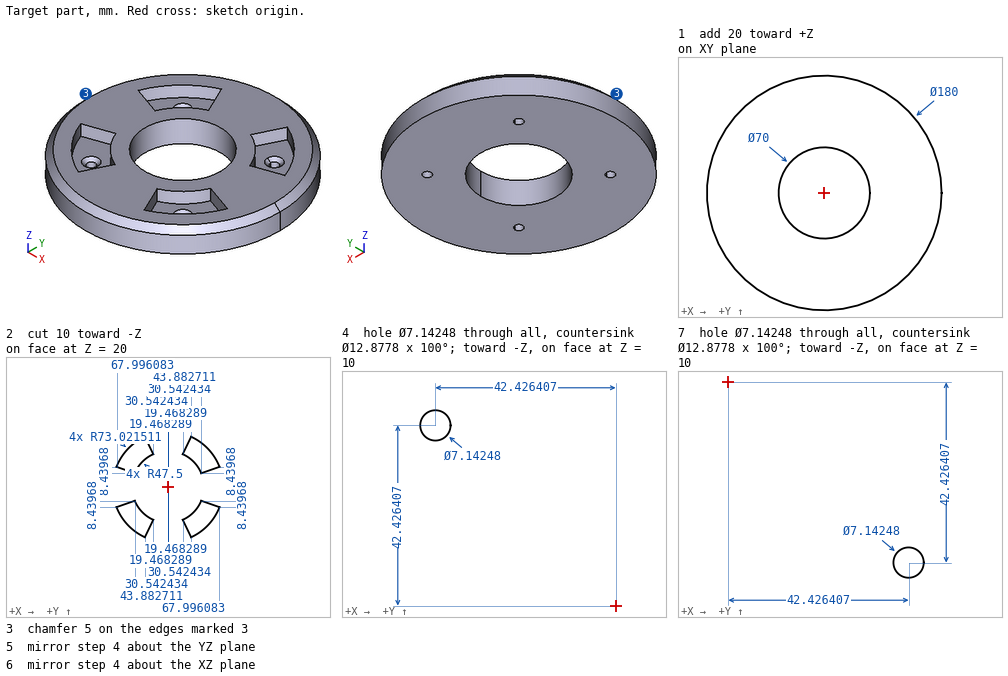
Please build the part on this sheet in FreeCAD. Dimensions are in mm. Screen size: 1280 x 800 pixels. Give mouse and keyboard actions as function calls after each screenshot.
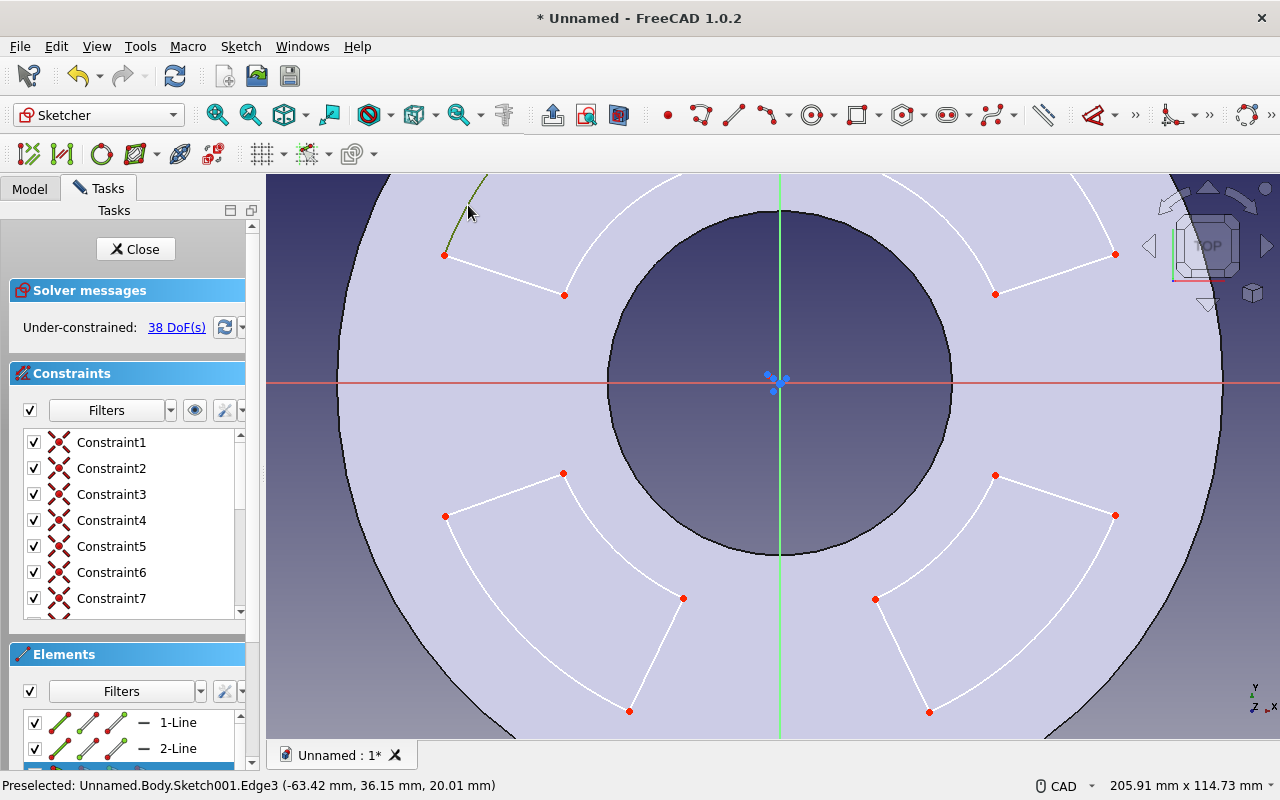
click(1091, 205)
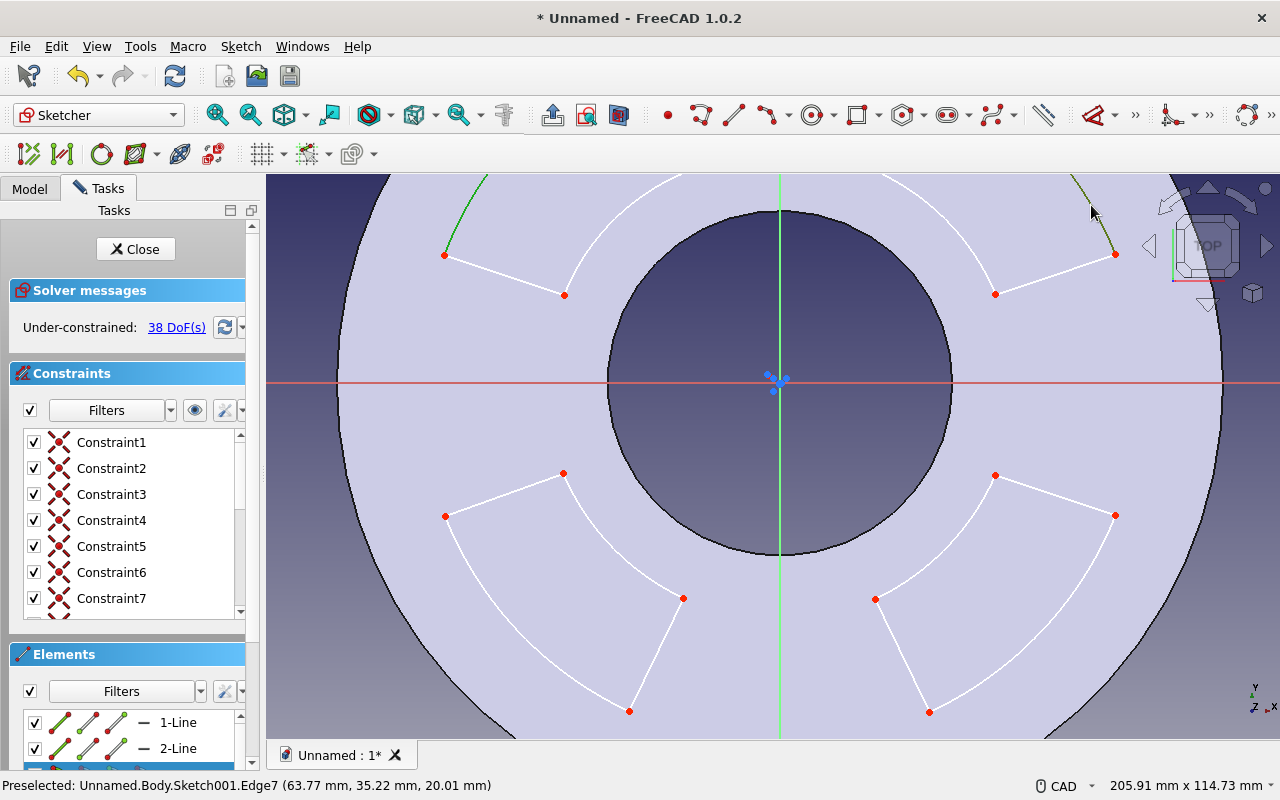
key(c)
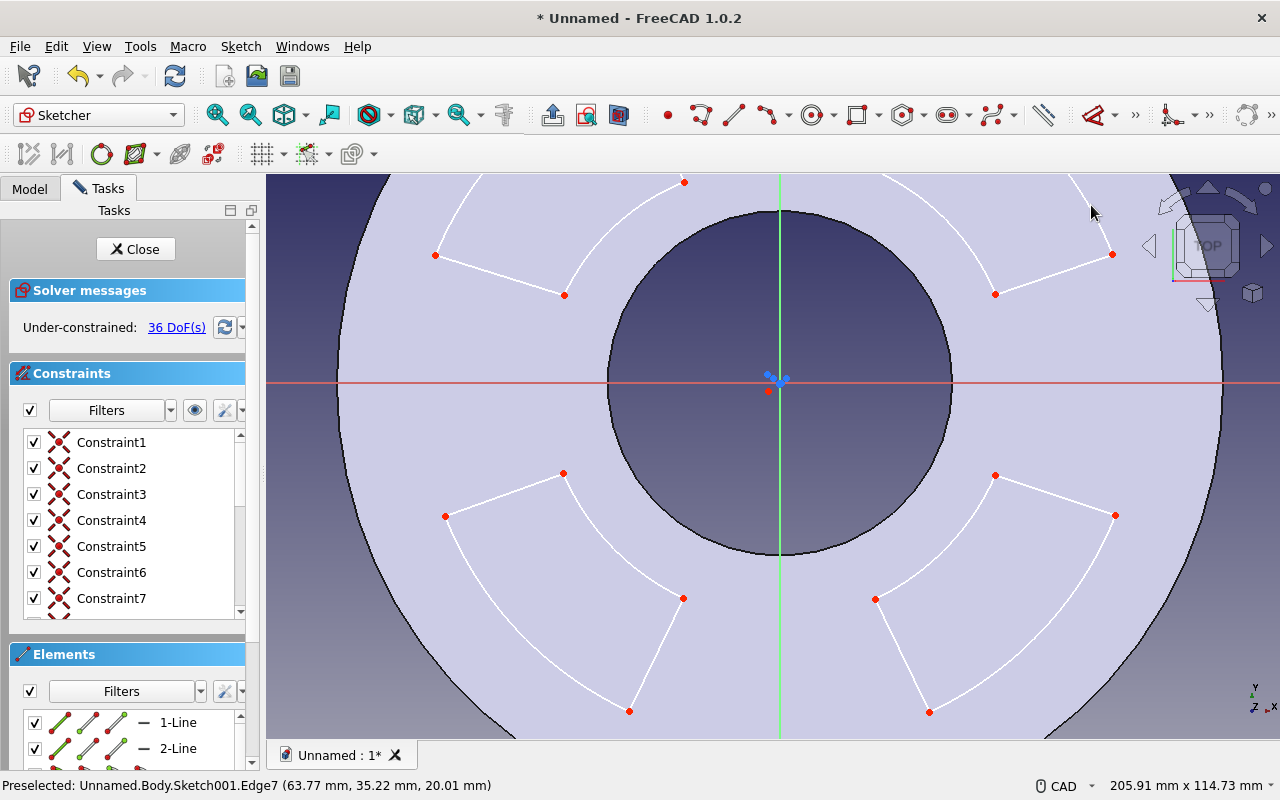
click(461, 205)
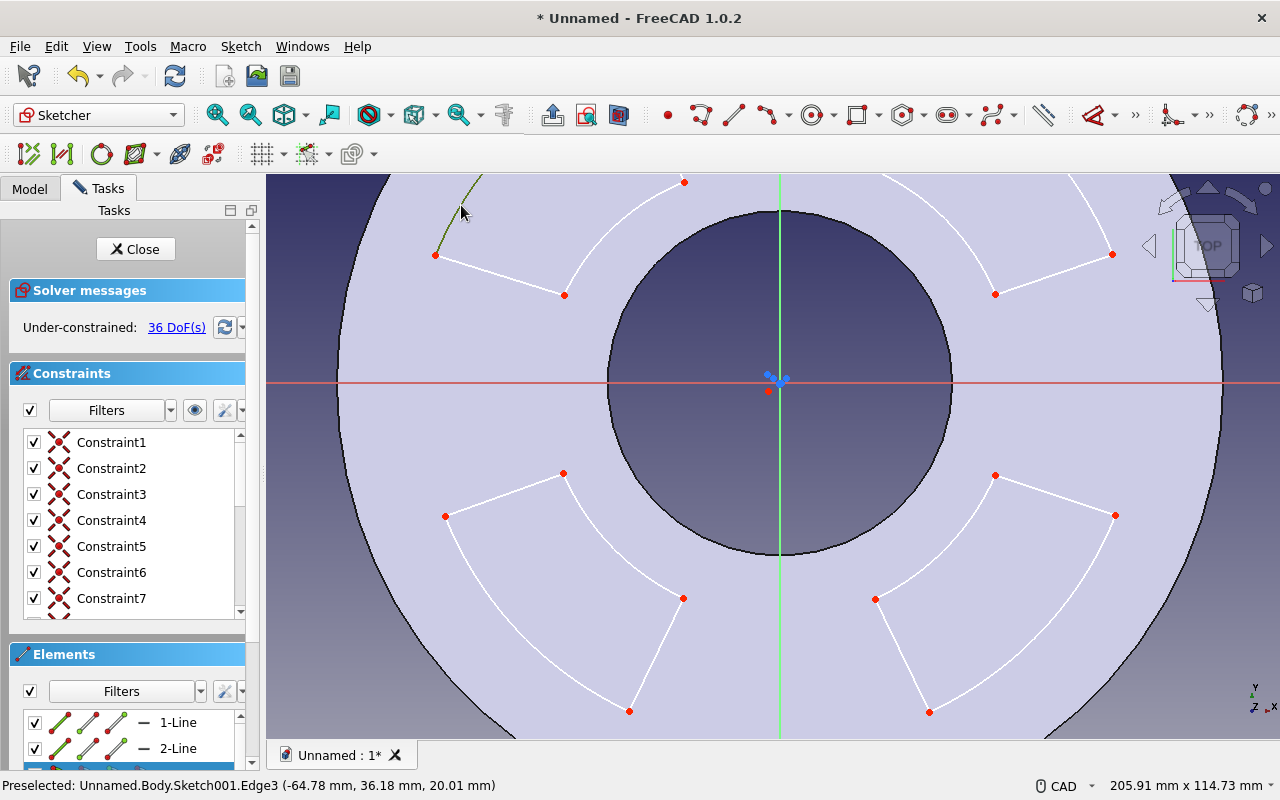
click(970, 248)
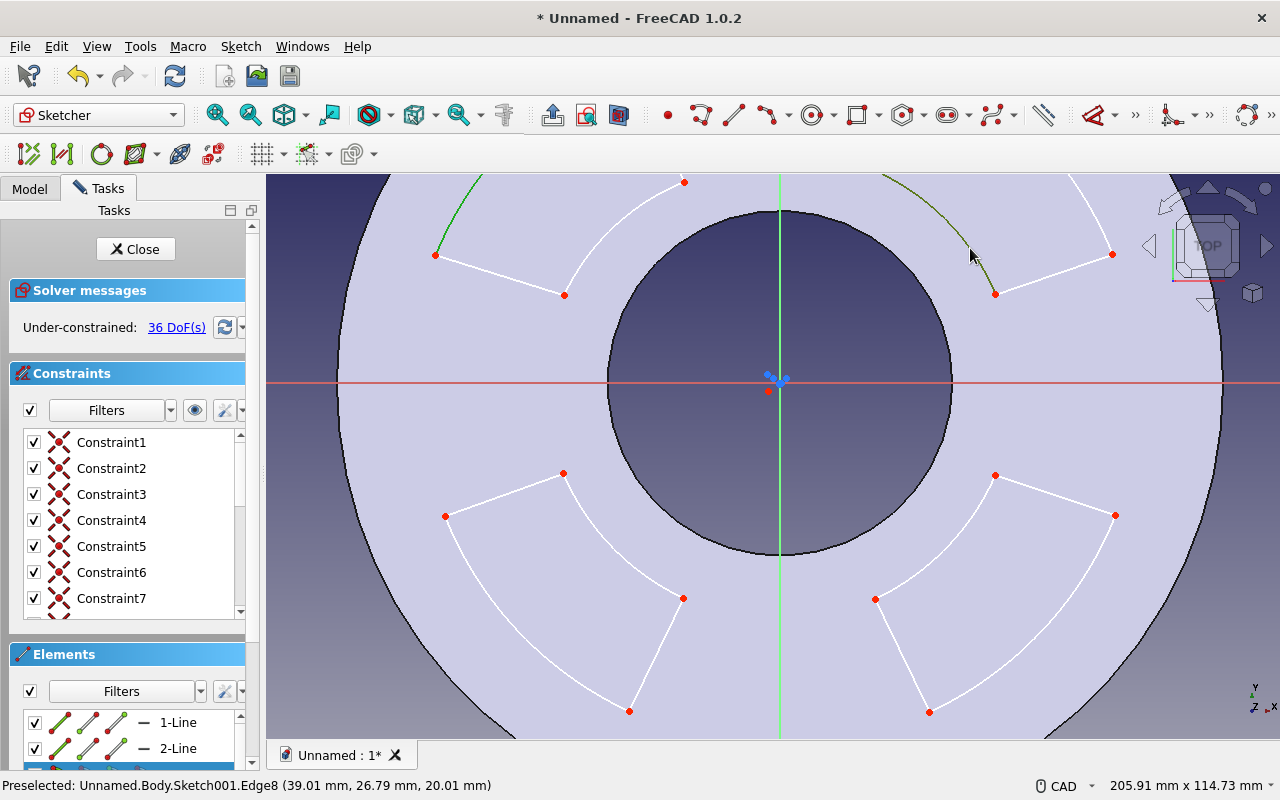
key(c)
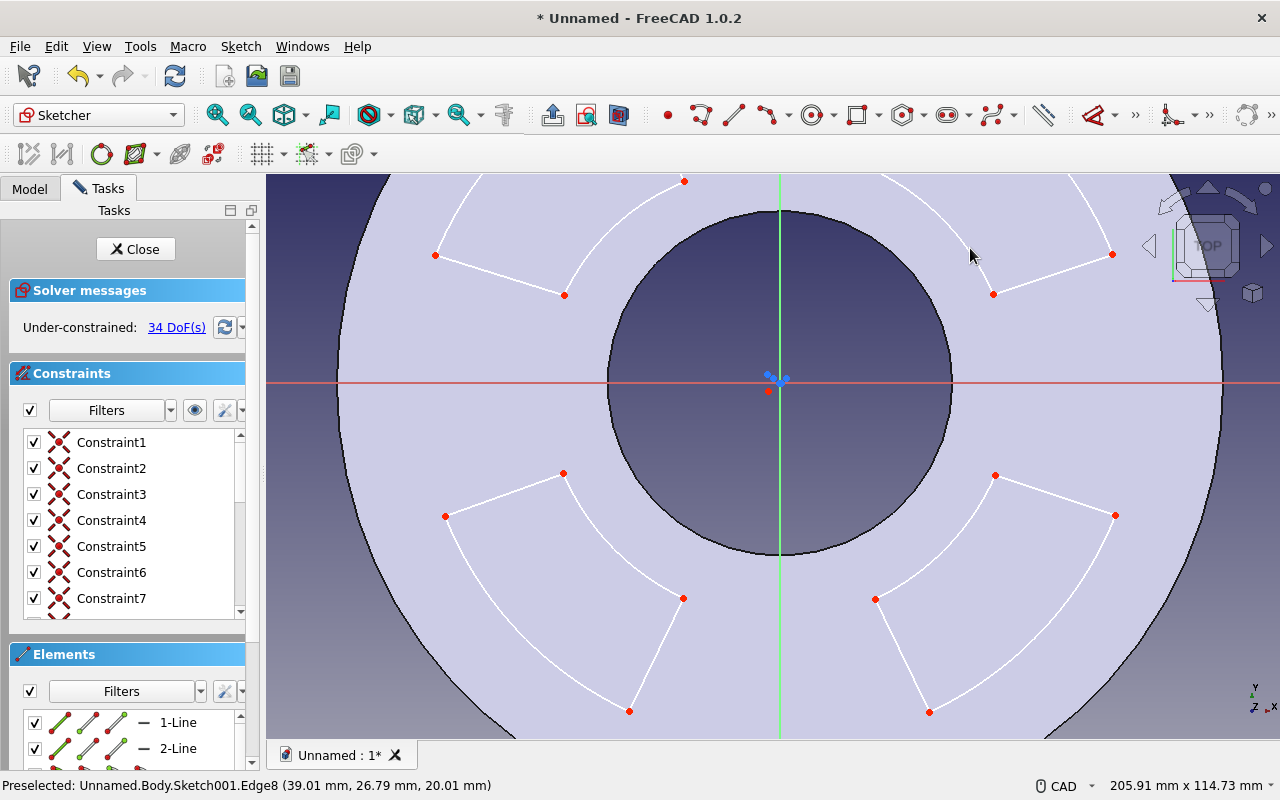
click(461, 205)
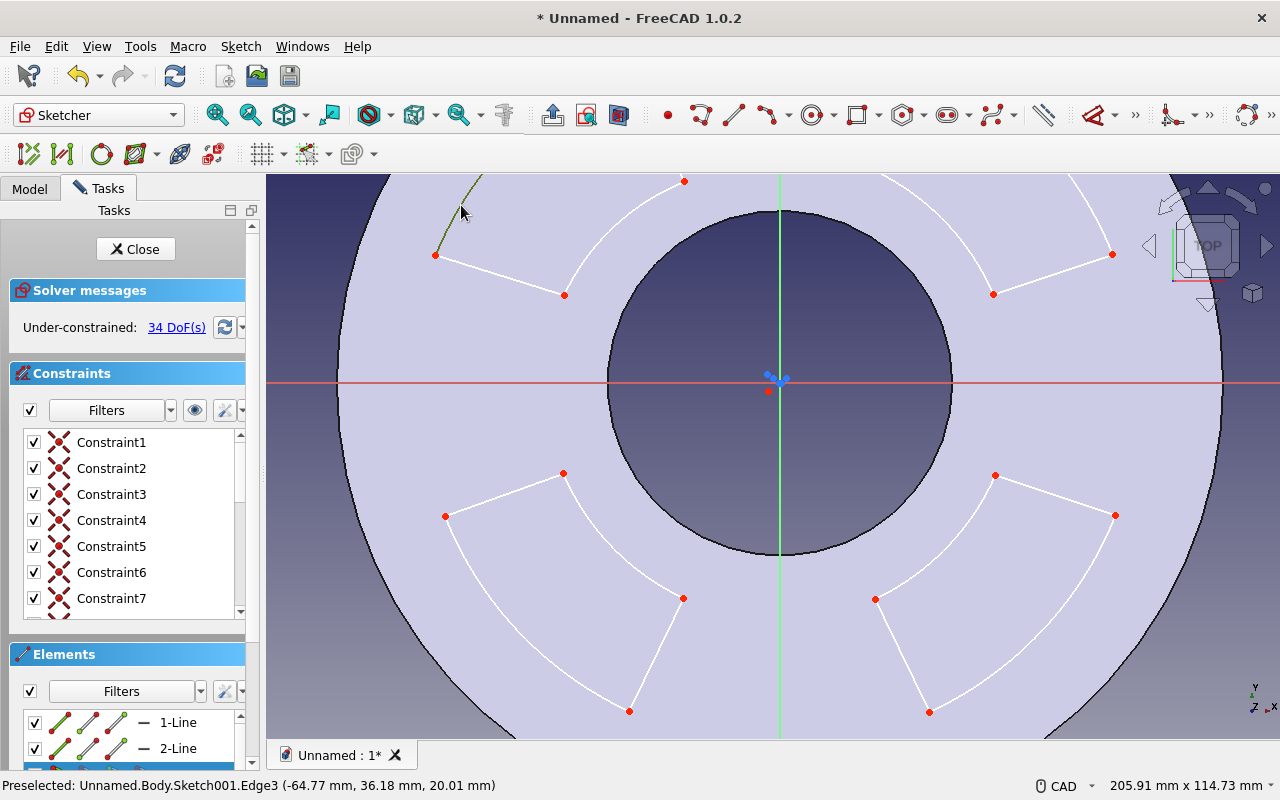
click(1000, 669)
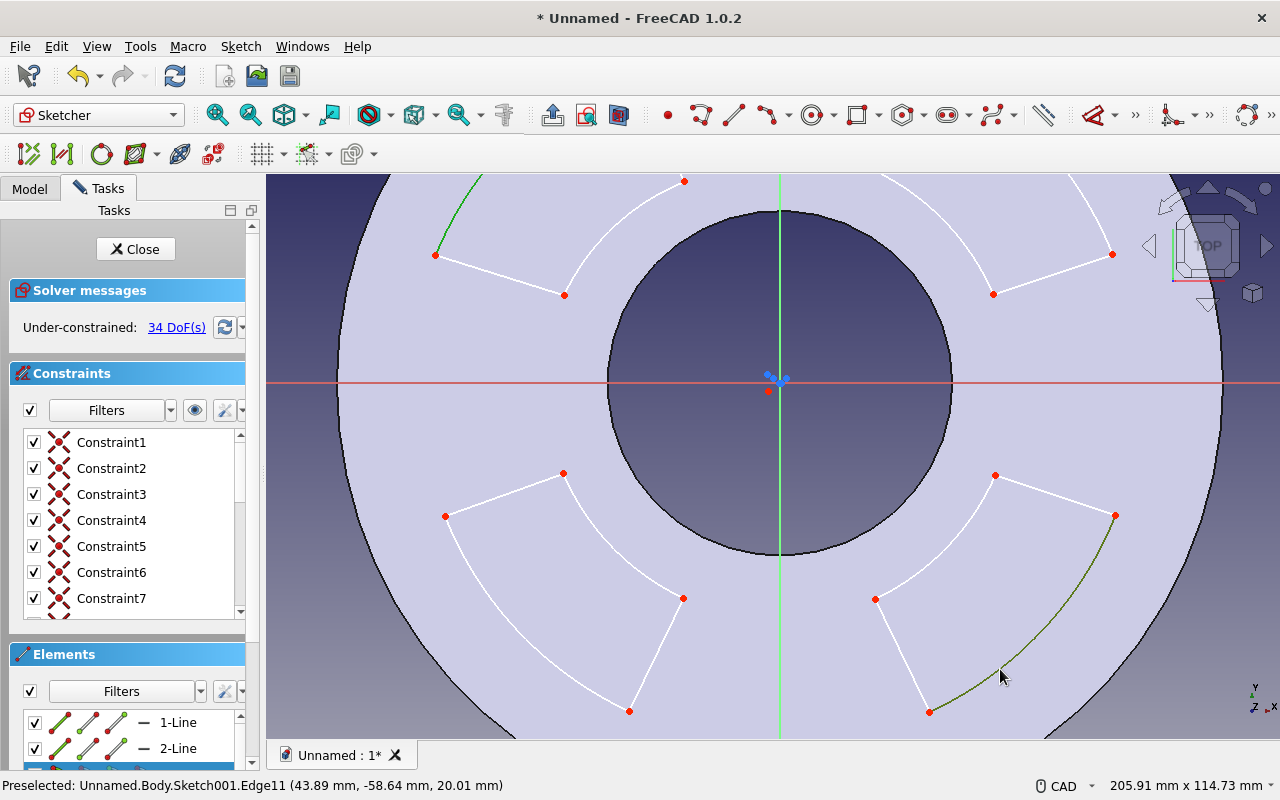
key(c)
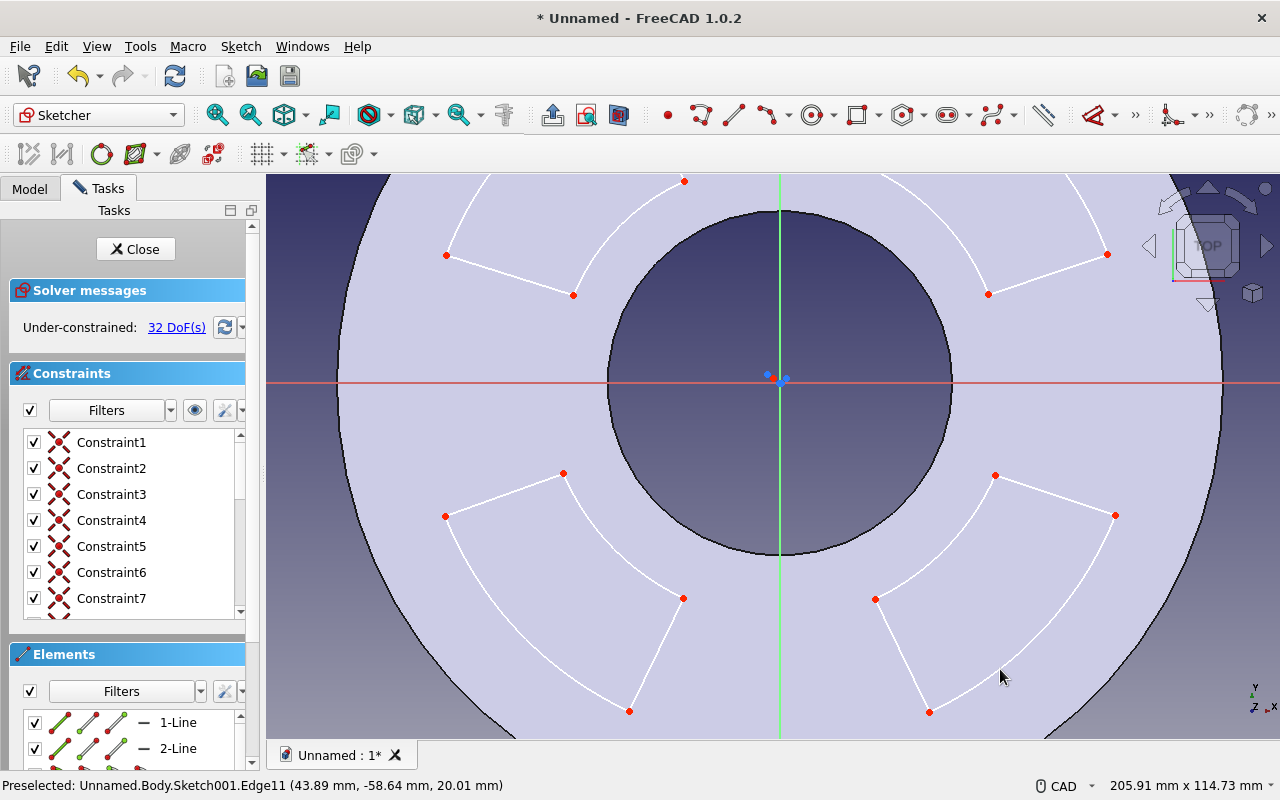
click(470, 206)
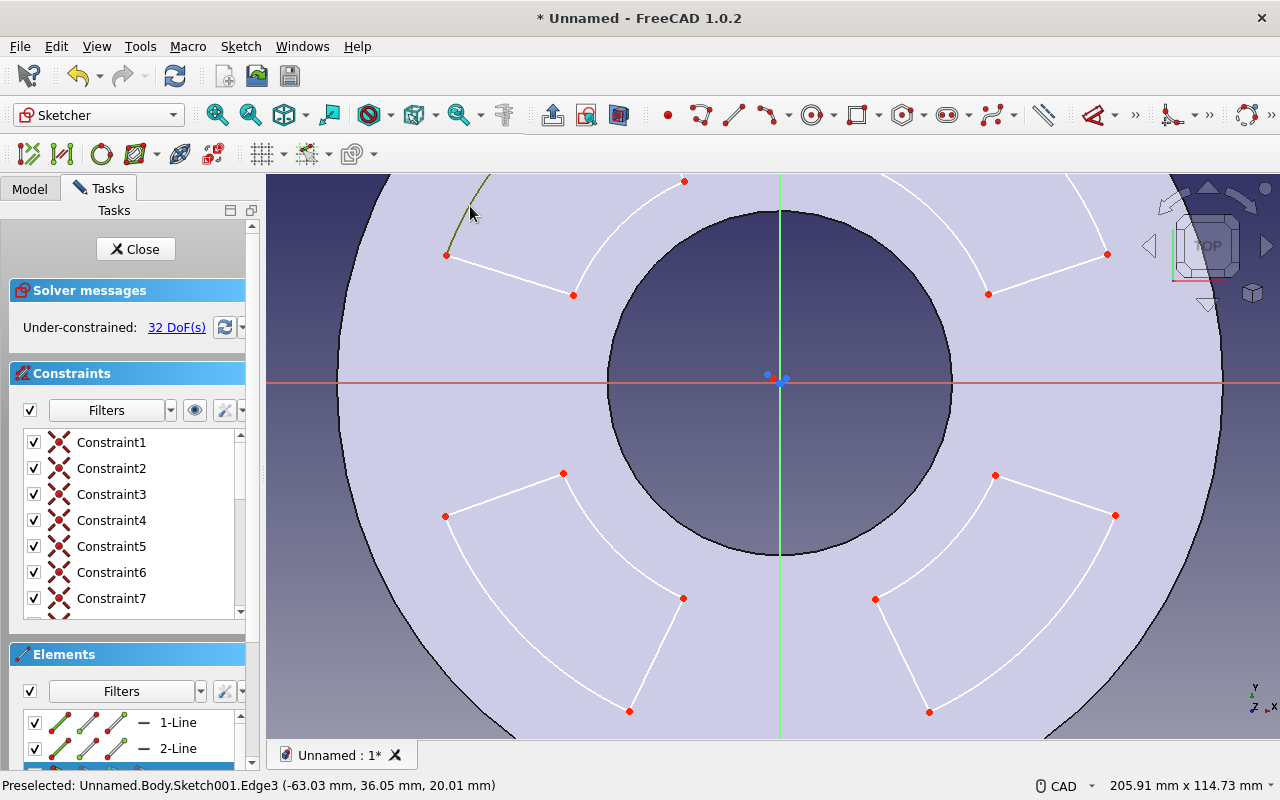
click(920, 571)